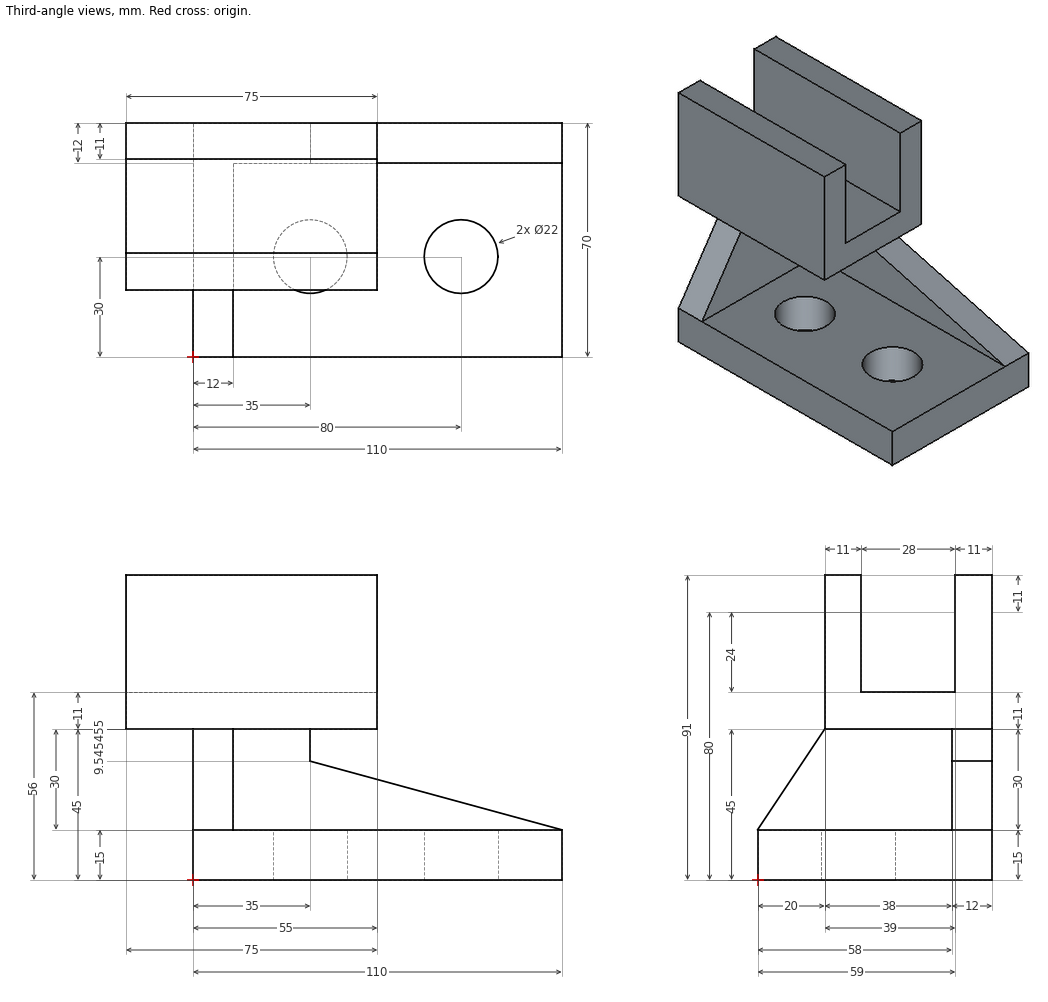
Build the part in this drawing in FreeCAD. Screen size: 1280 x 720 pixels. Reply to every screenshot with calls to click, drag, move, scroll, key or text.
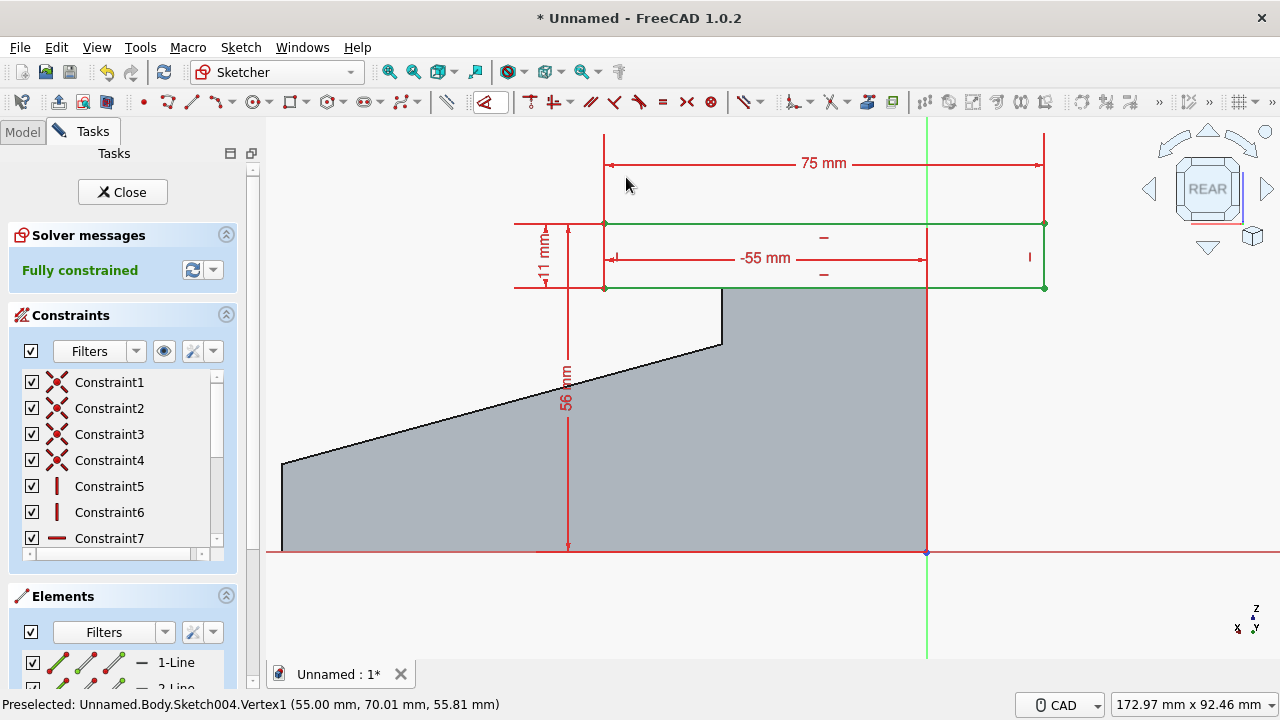
click(123, 192)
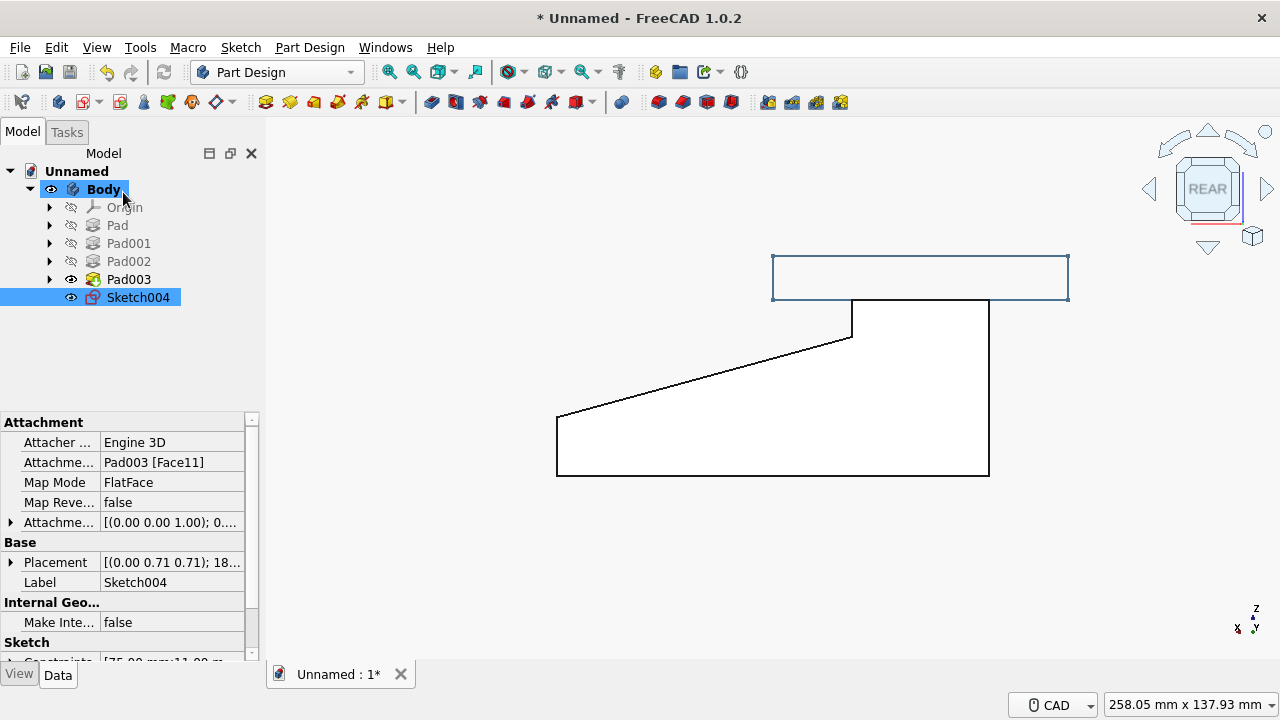
click(266, 102)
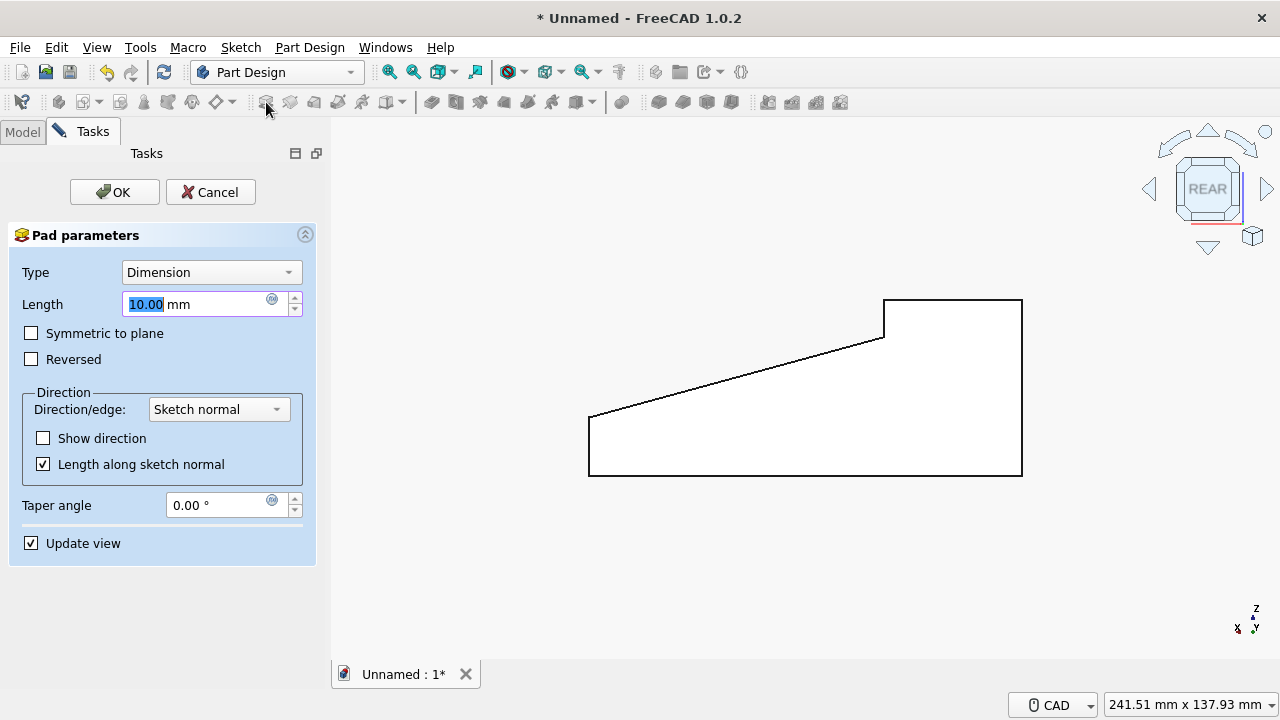
text(11)
key(Tab)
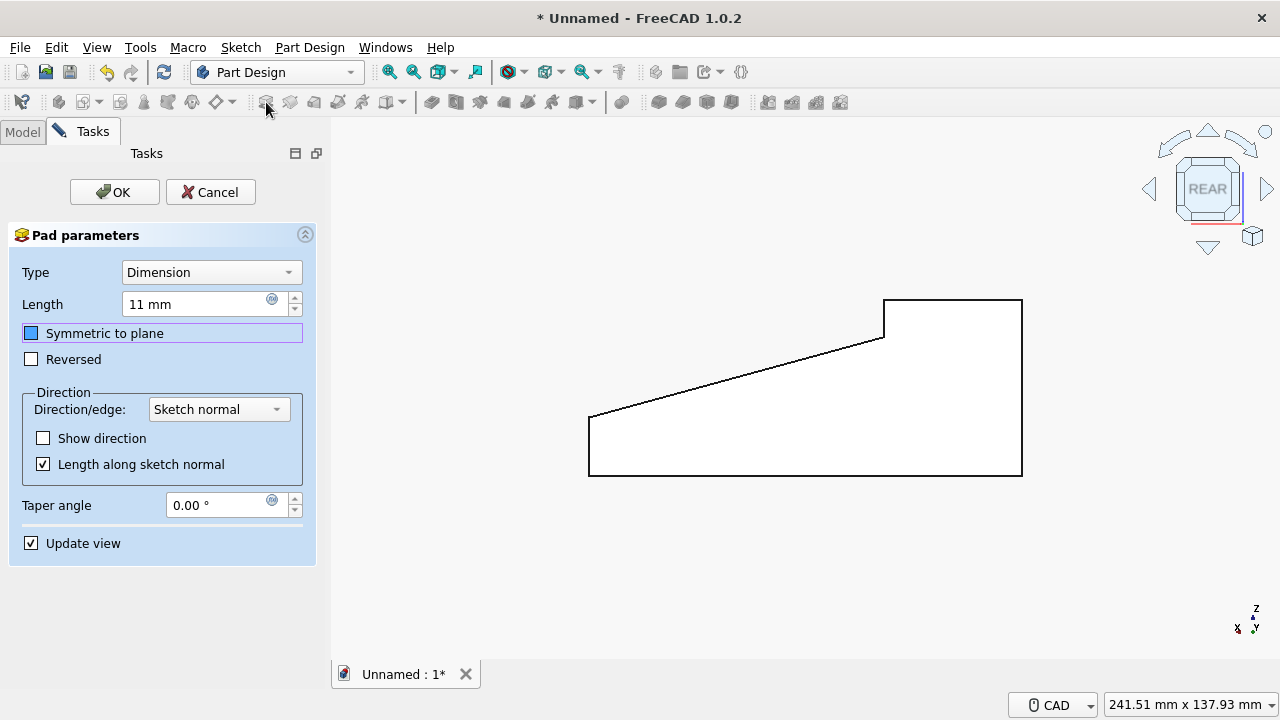
click(30, 359)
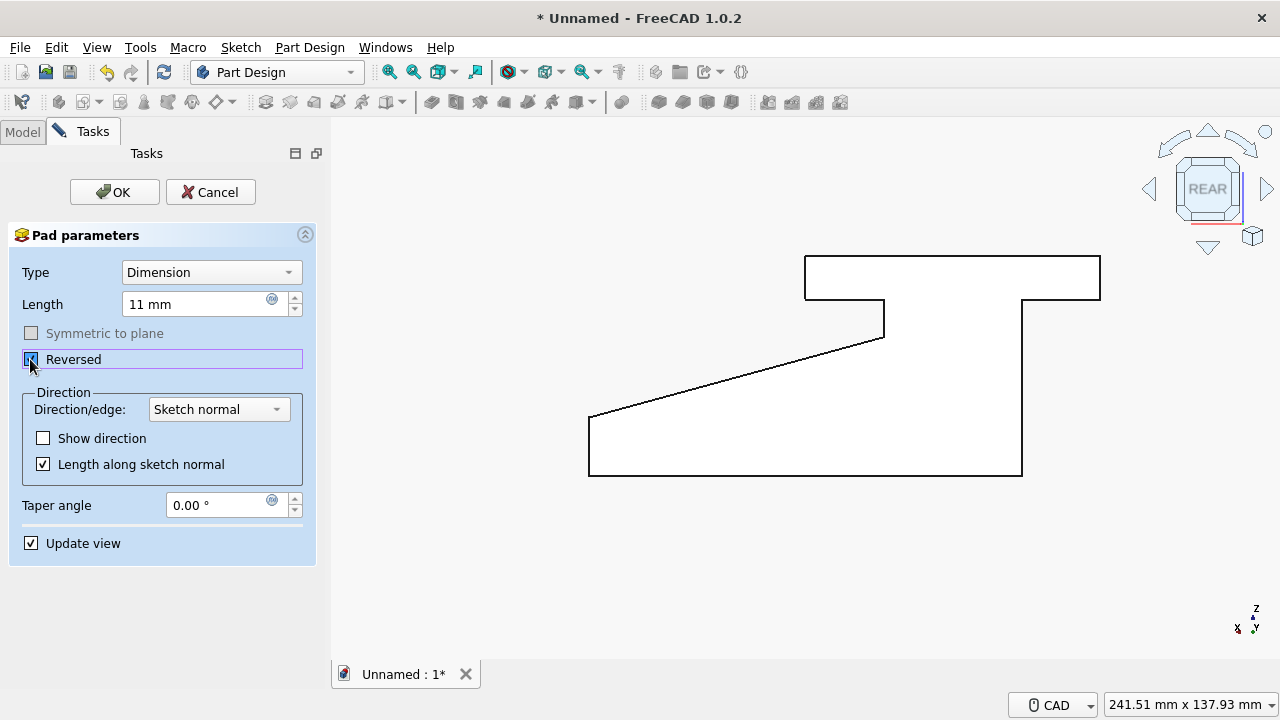
click(115, 192)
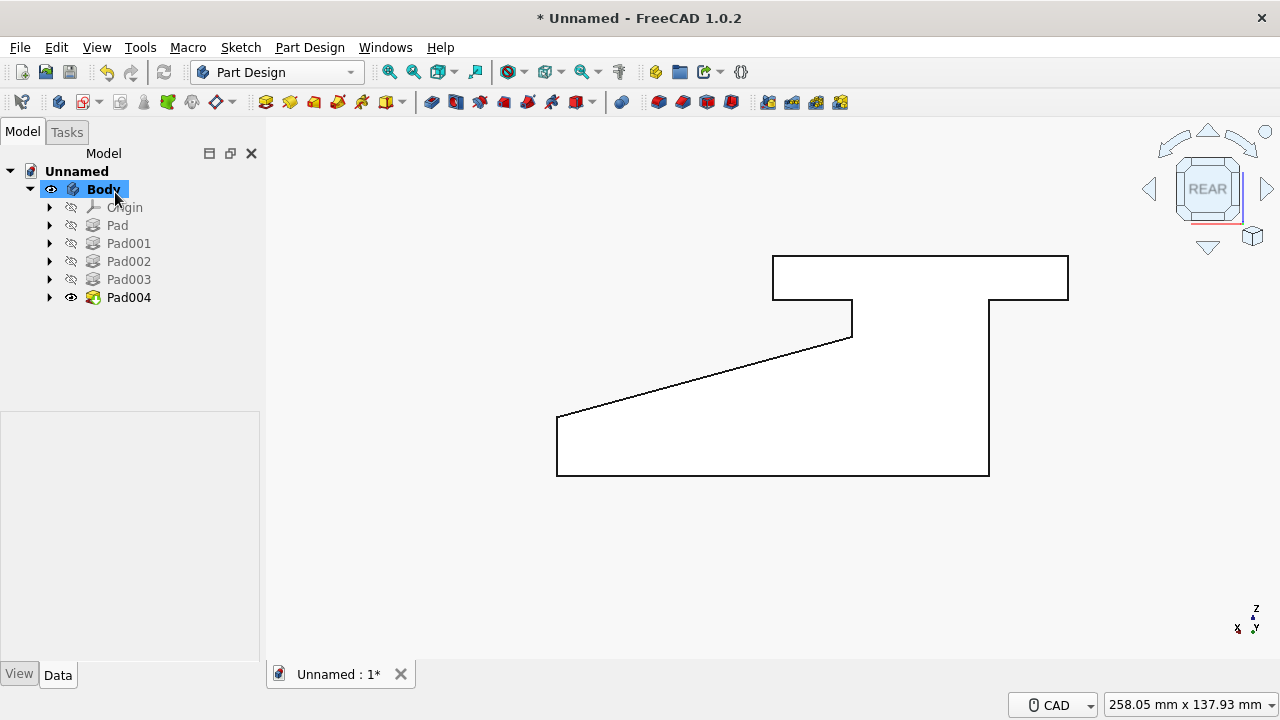
key(0)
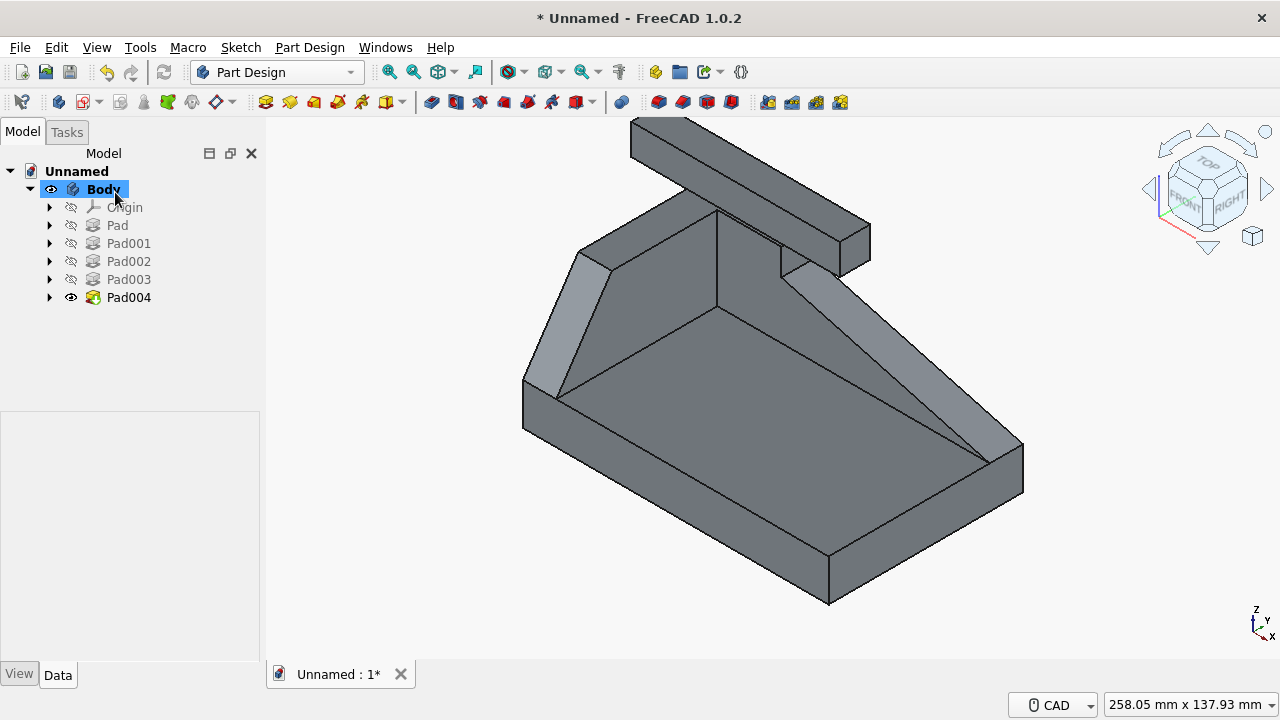
key(v)
key(f)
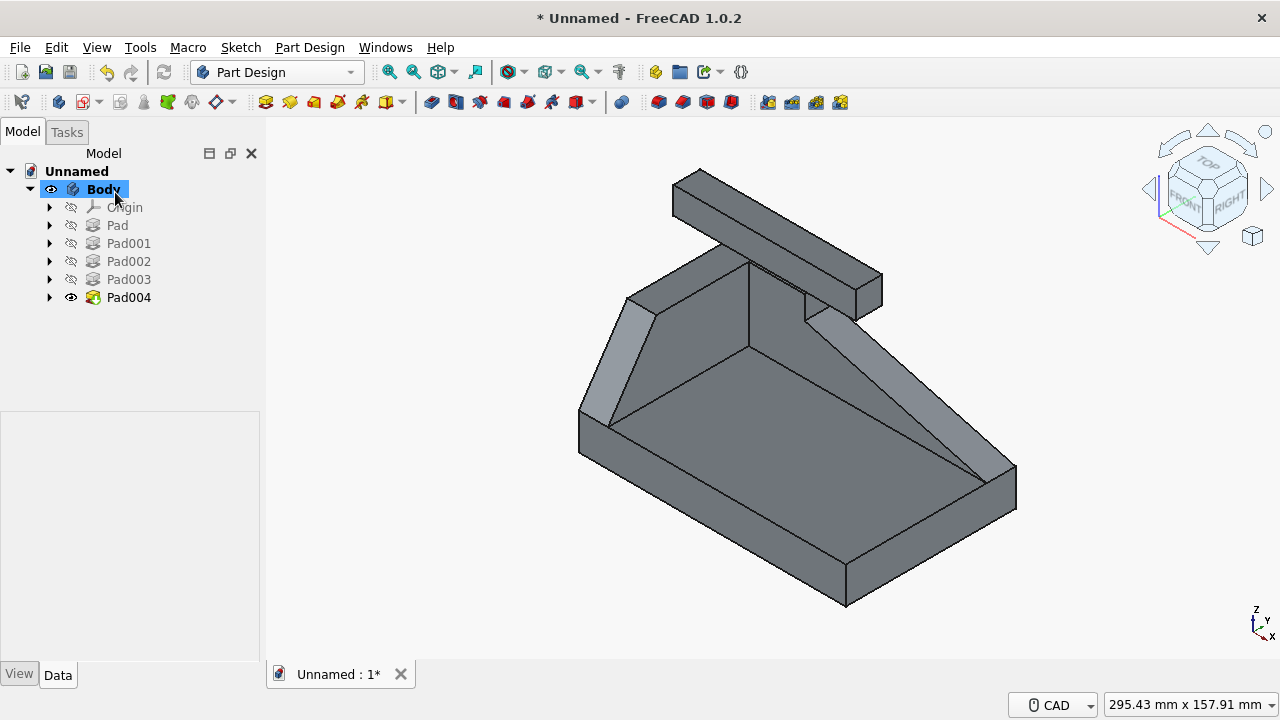
click(869, 297)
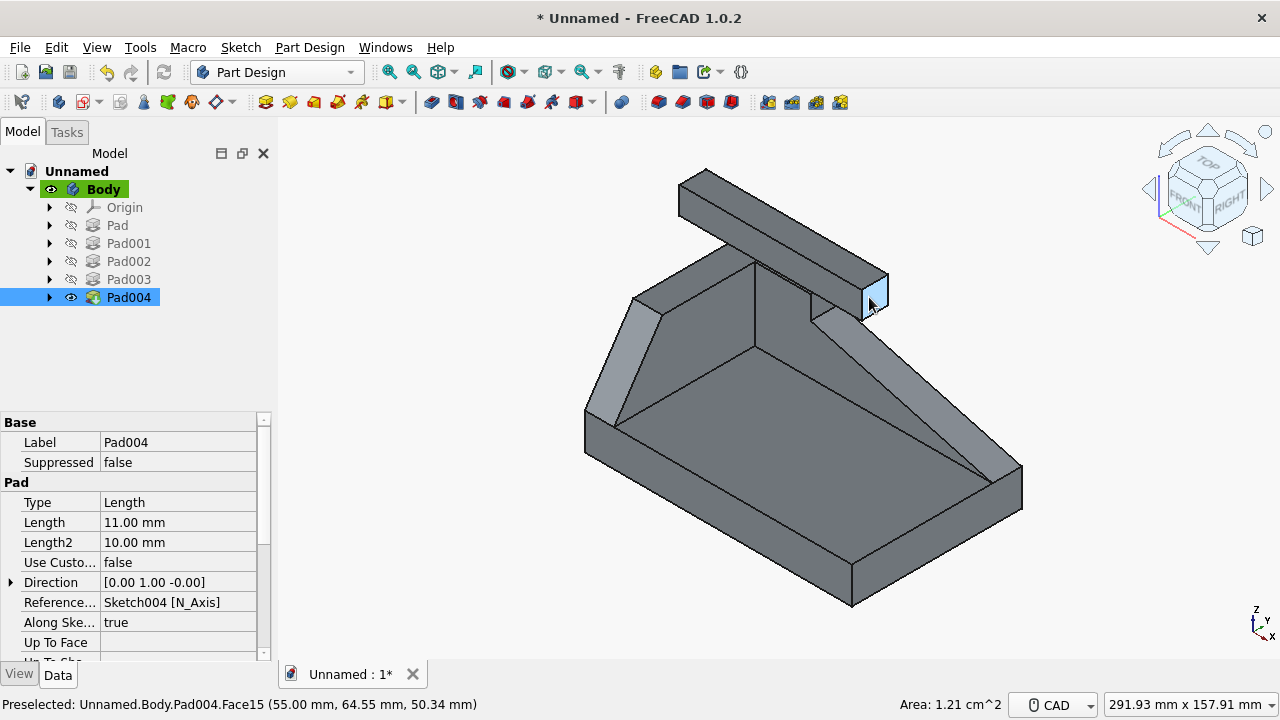
click(84, 102)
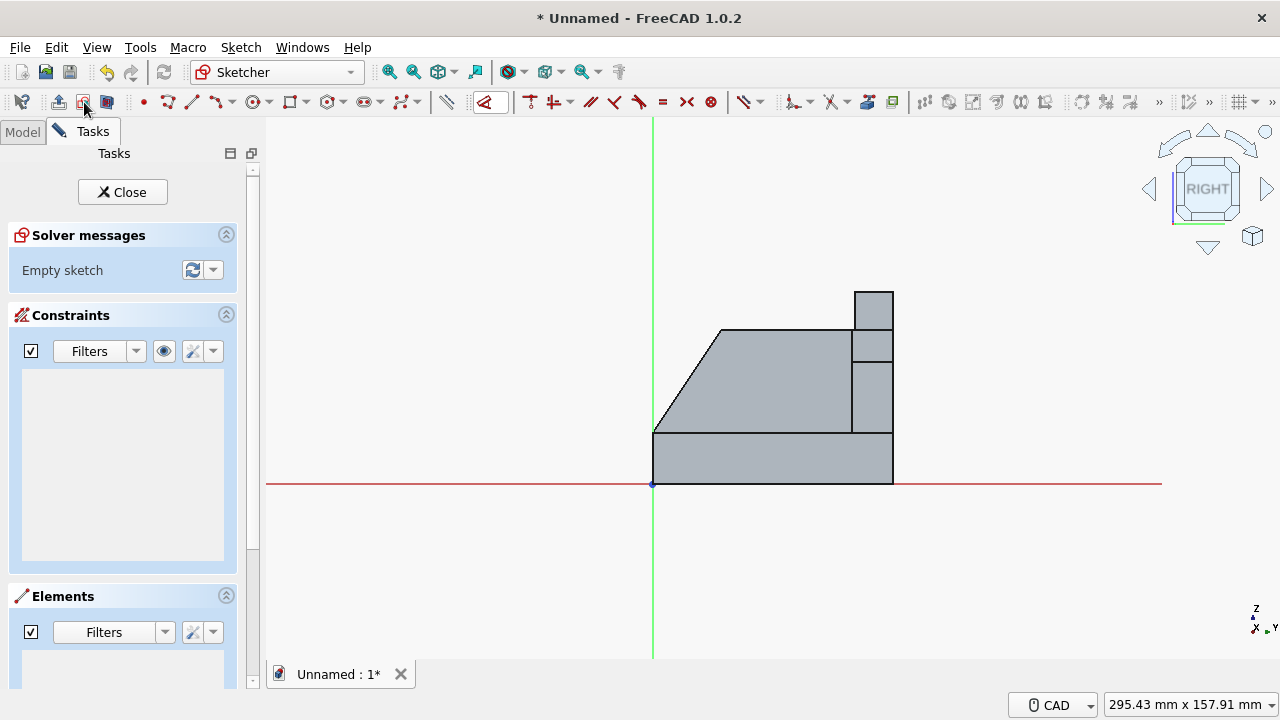
click(108, 102)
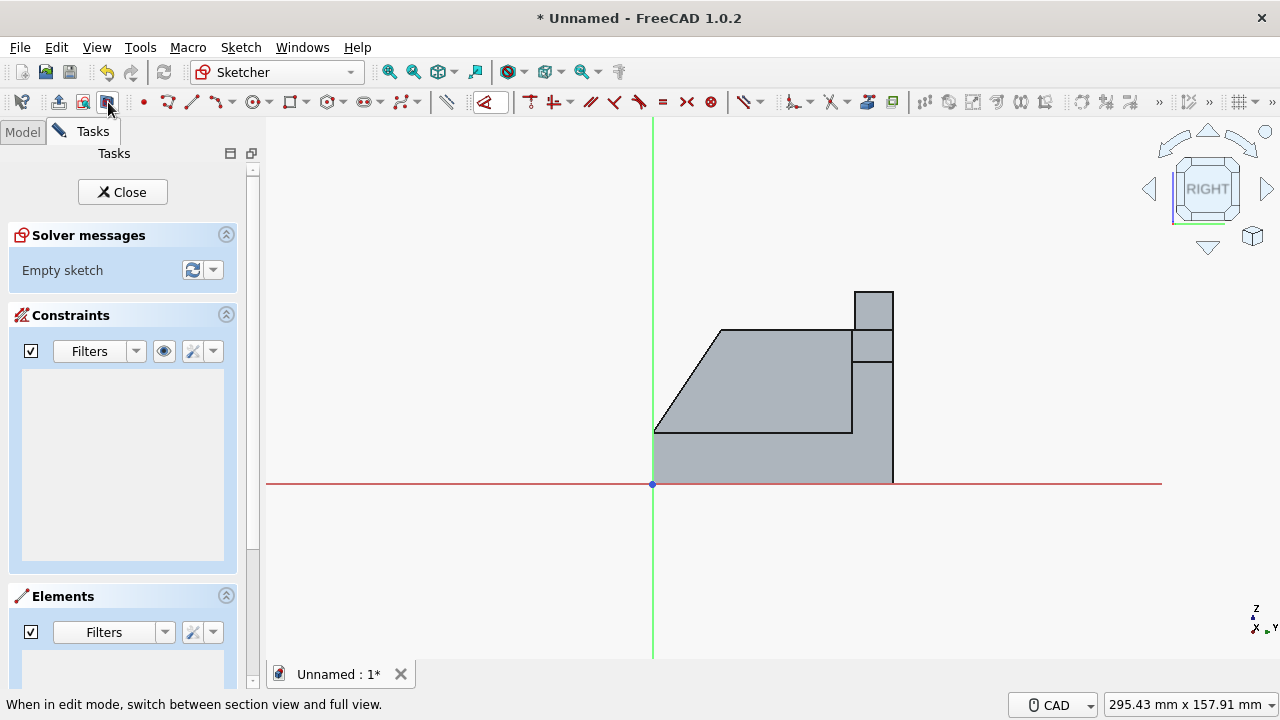
click(168, 102)